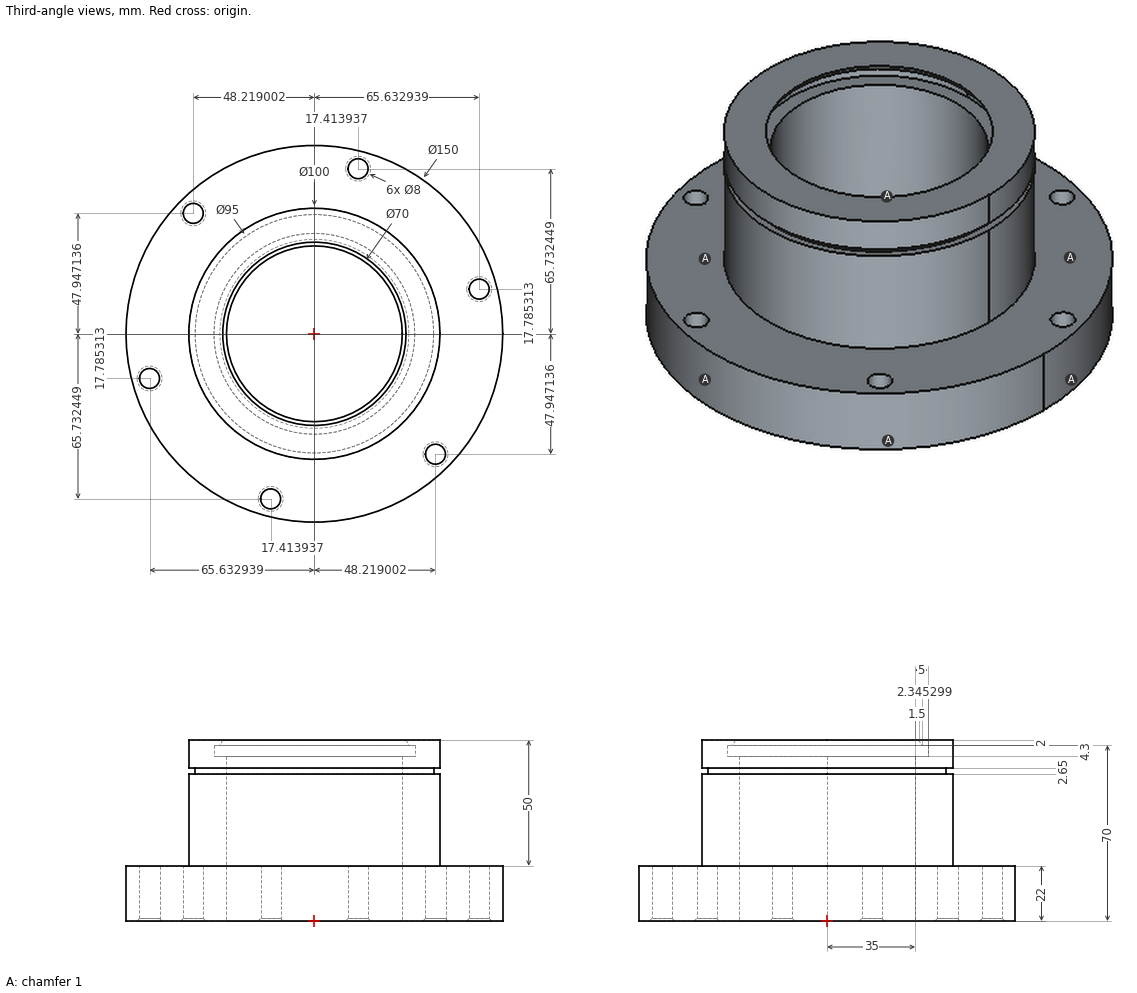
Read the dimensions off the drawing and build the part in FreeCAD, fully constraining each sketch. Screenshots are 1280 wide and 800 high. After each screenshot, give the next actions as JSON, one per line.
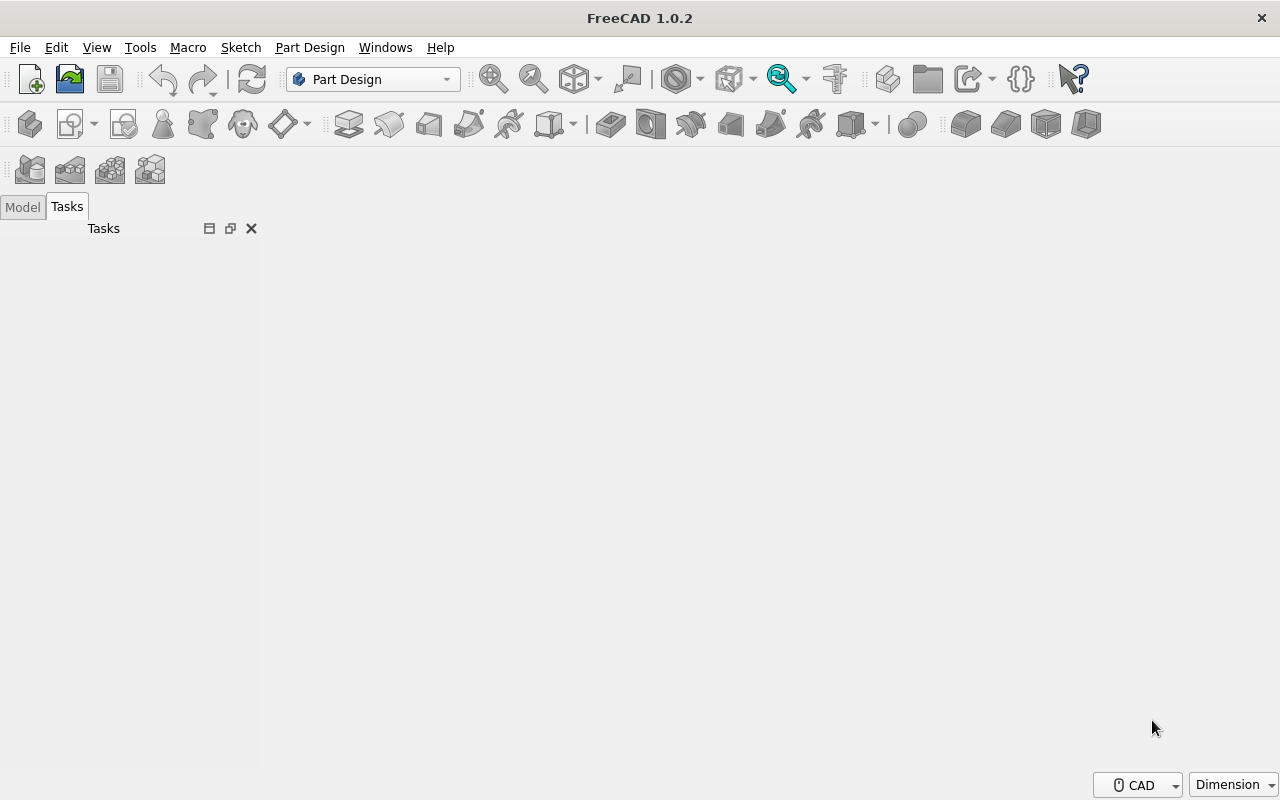
{"action": "left_click", "coordinate": [30, 80]}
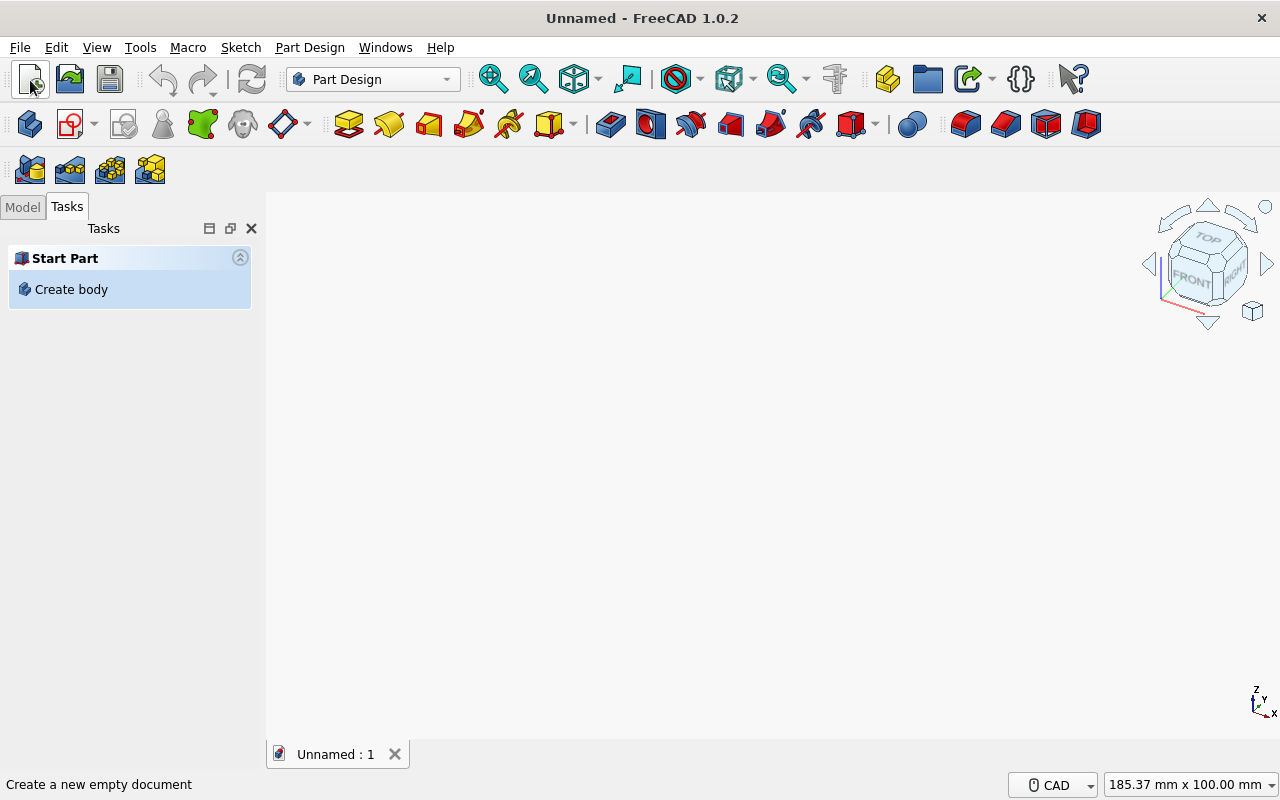
{"action": "left_click", "coordinate": [70, 124]}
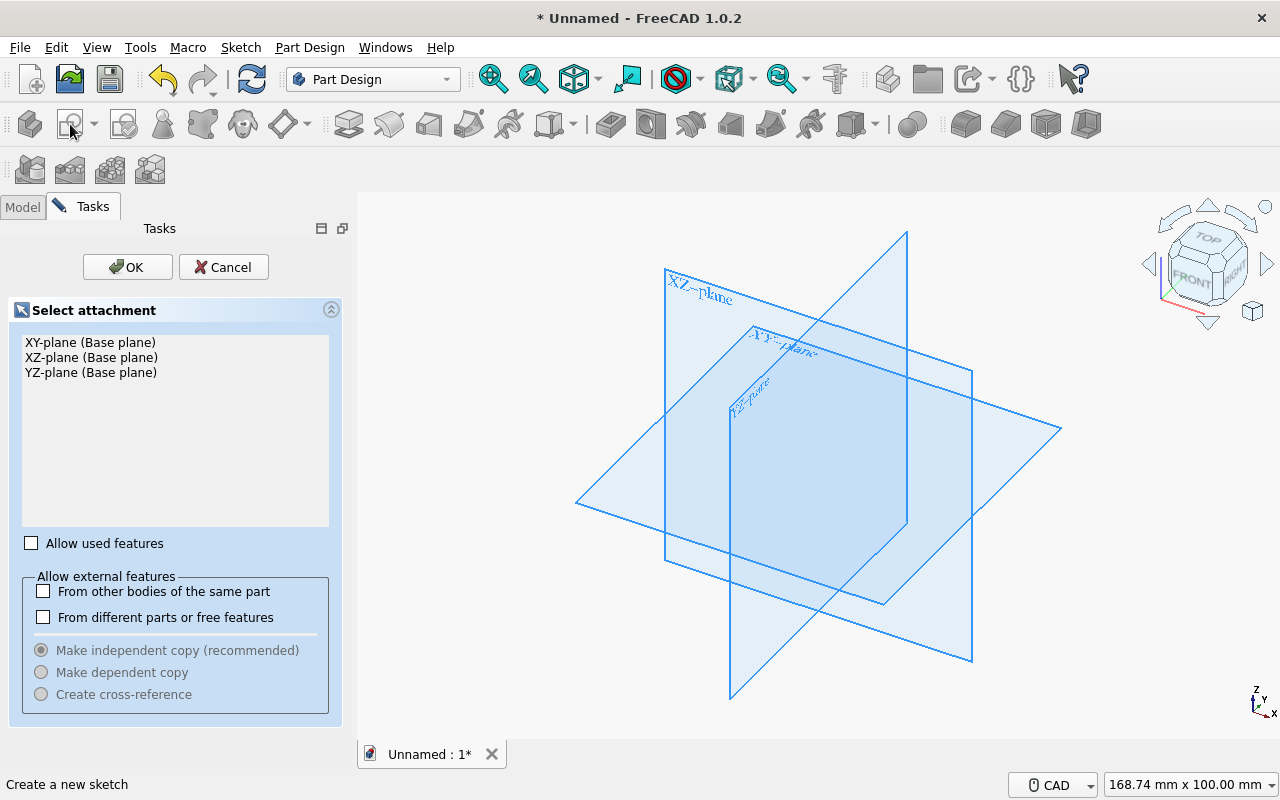
{"action": "left_click", "coordinate": [82, 342]}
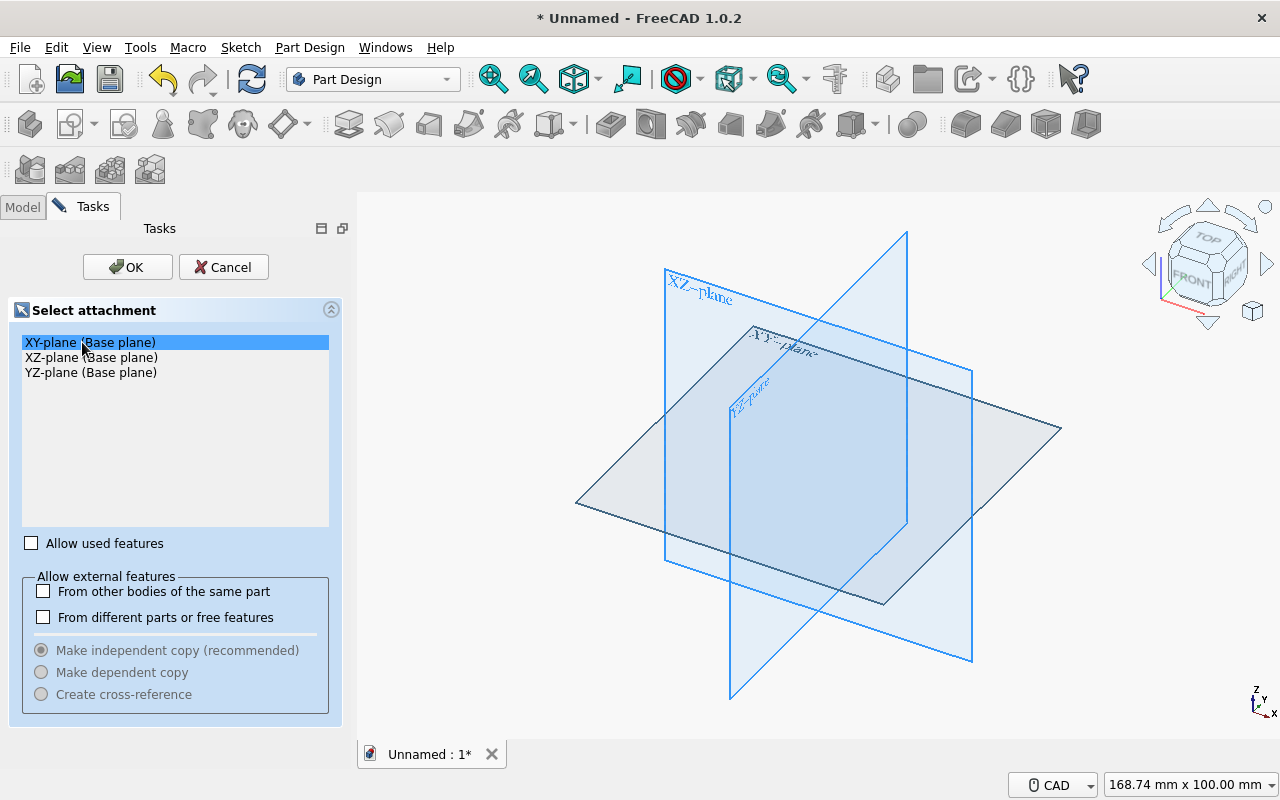
{"action": "left_click", "coordinate": [128, 267]}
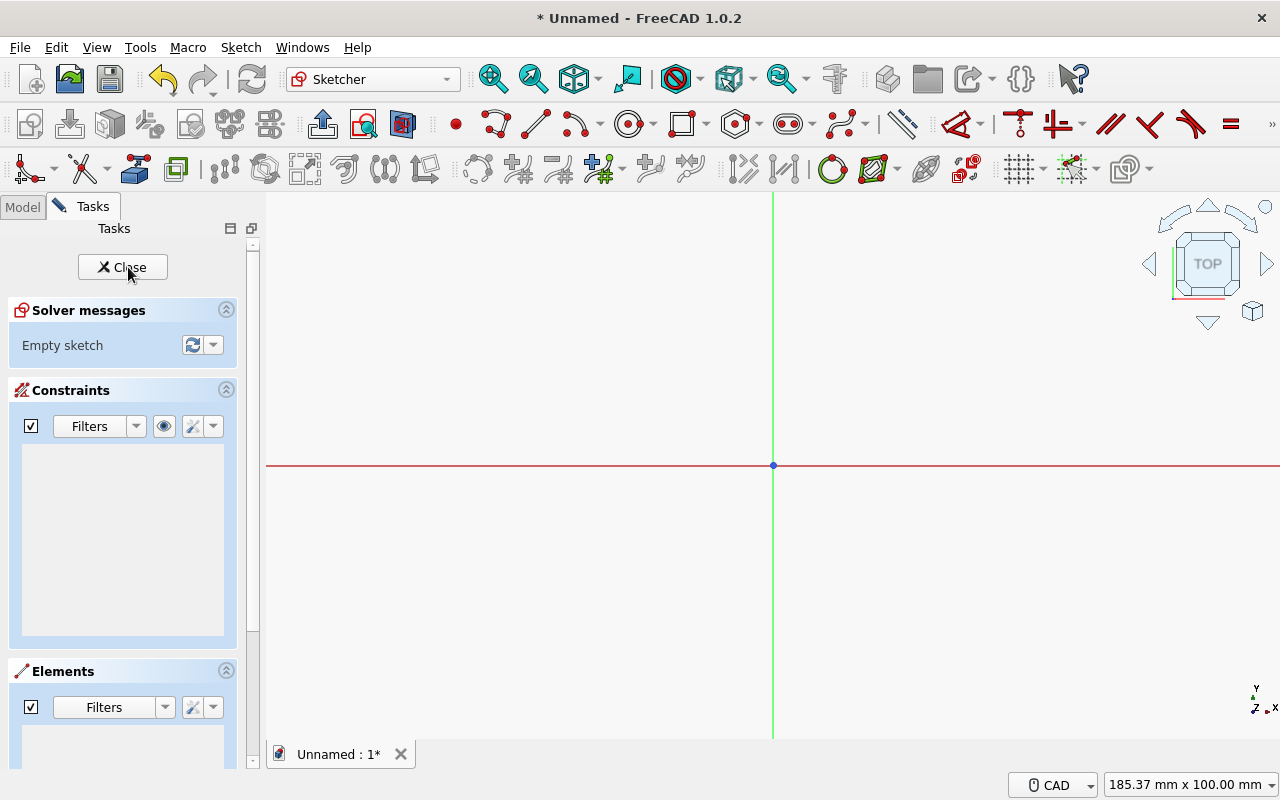
{"action": "scroll", "coordinate": [649, 466], "scroll_direction": "down", "scroll_amount": 4}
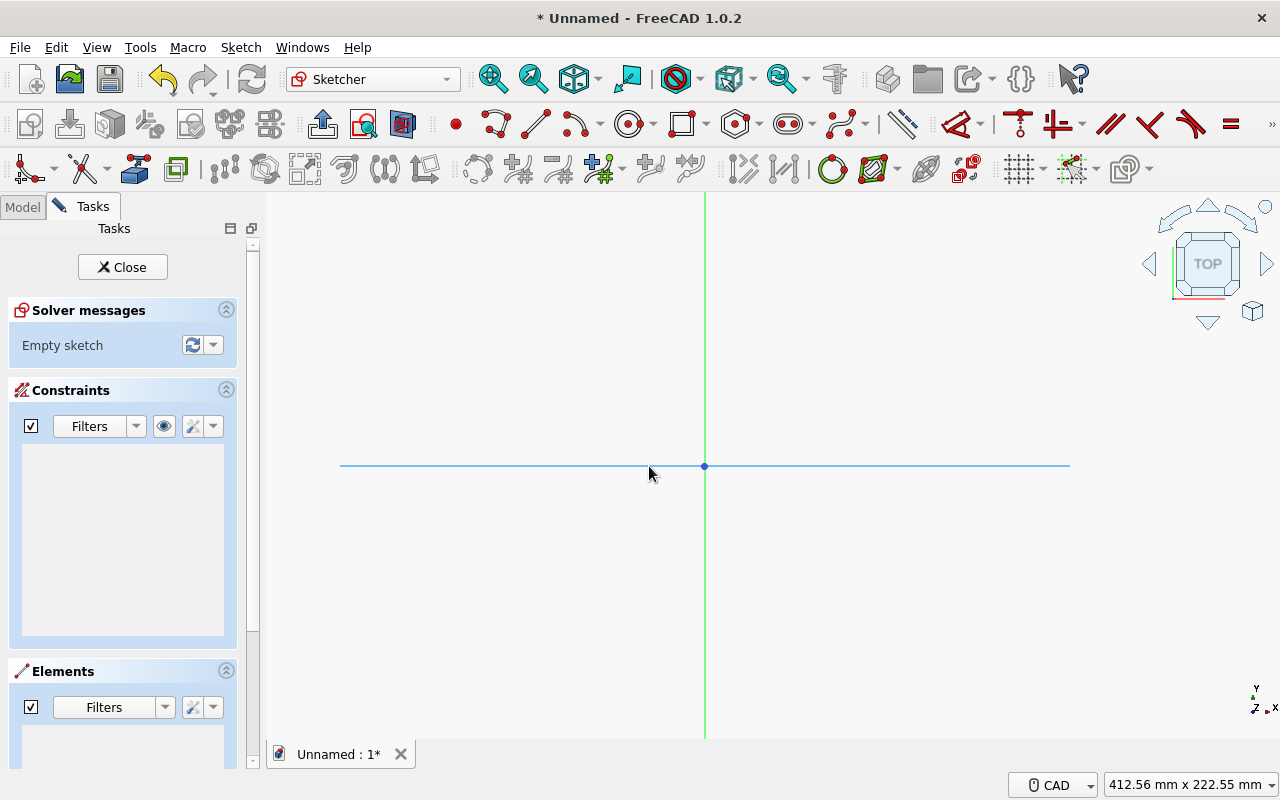
{"action": "left_click", "coordinate": [630, 124]}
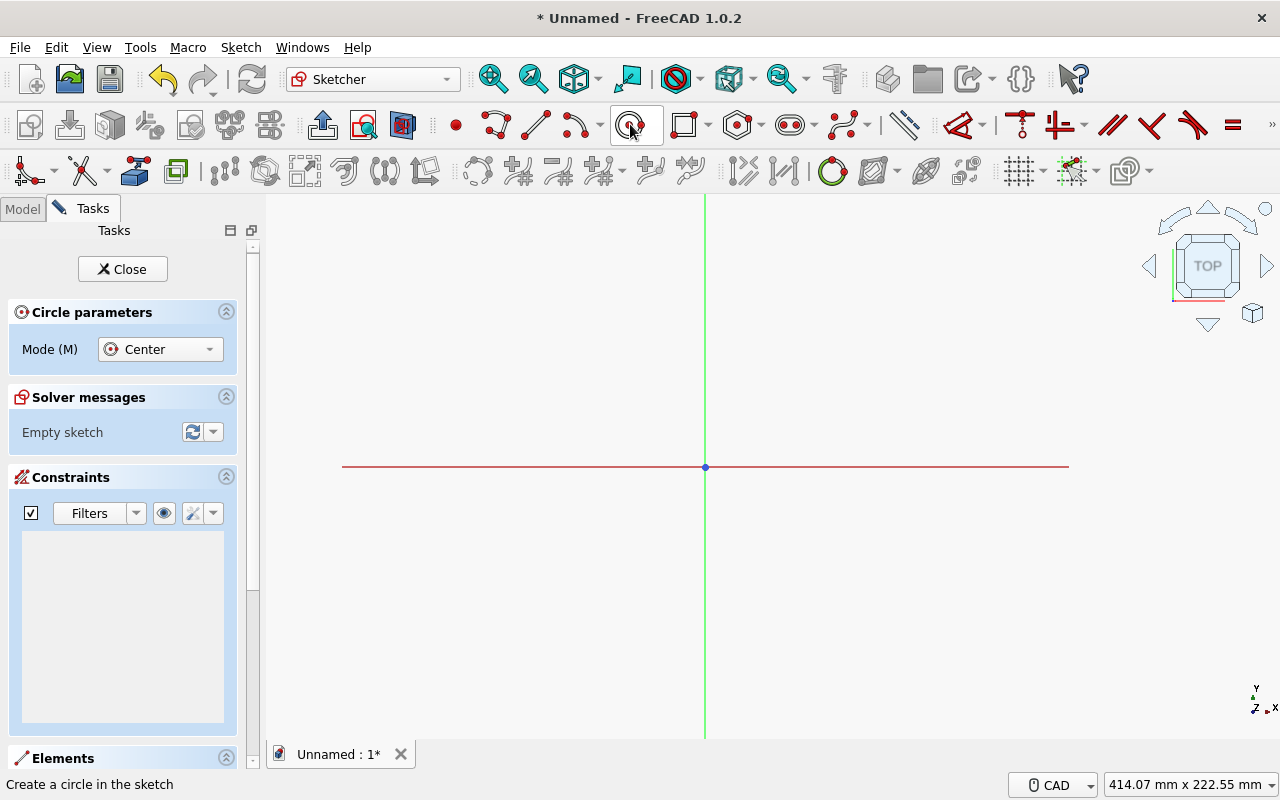
{"action": "left_click", "coordinate": [705, 467]}
{"action": "left_click", "coordinate": [835, 337]}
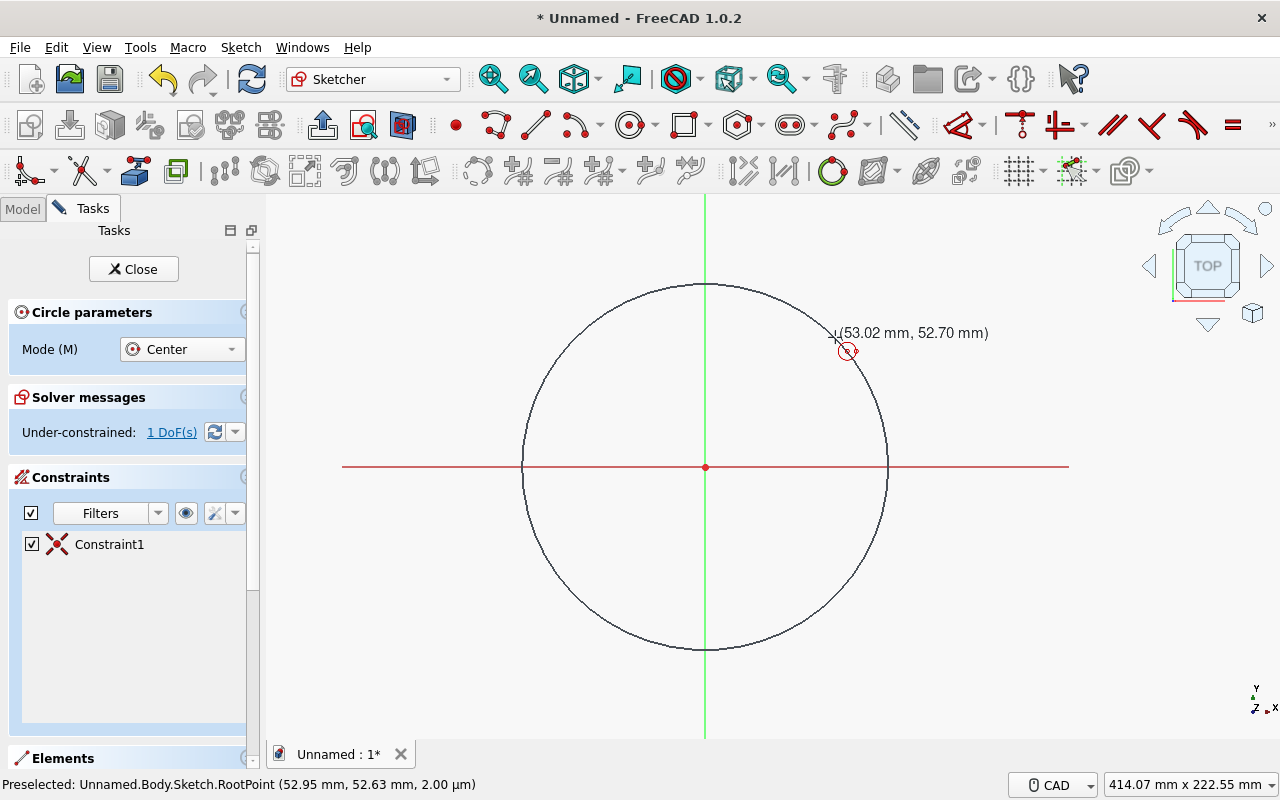
{"action": "left_click", "coordinate": [705, 467]}
{"action": "left_click", "coordinate": [766, 406]}
{"action": "key", "text": "Escape"}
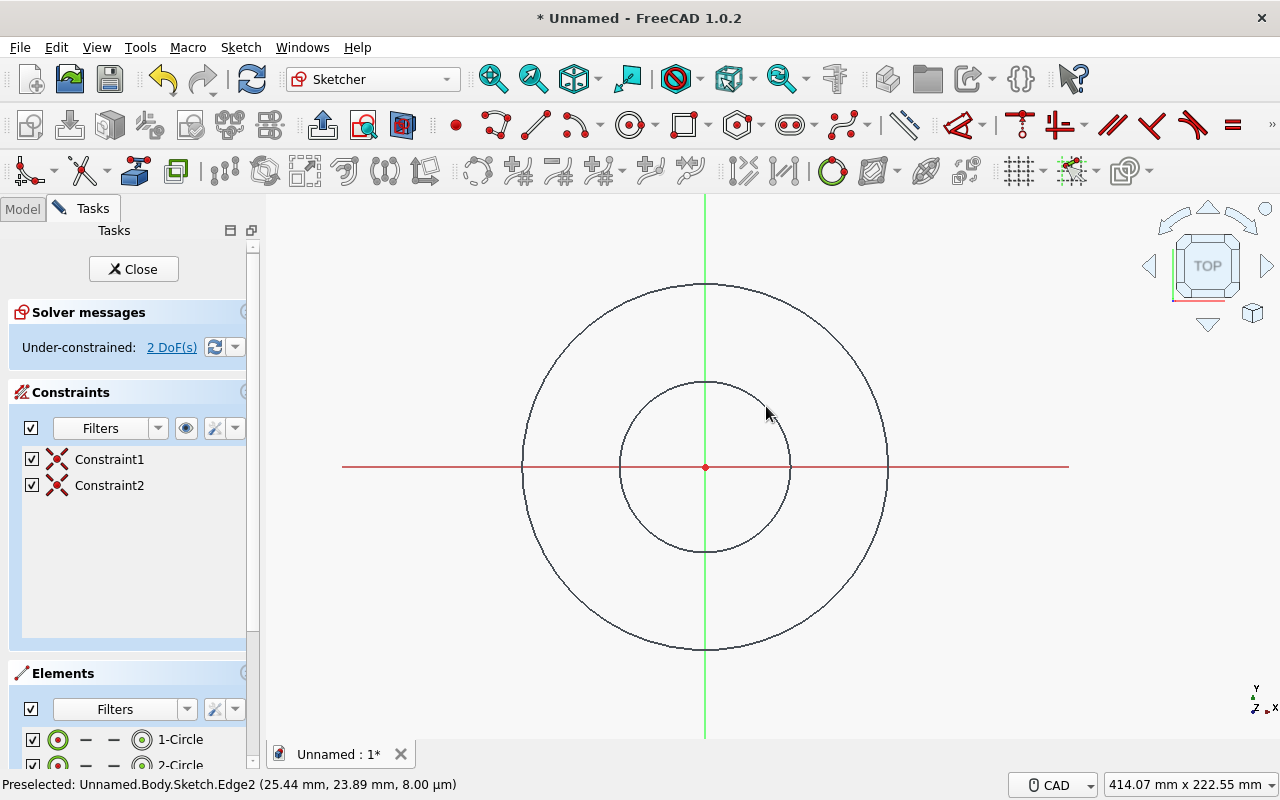
{"action": "left_click", "coordinate": [958, 126]}